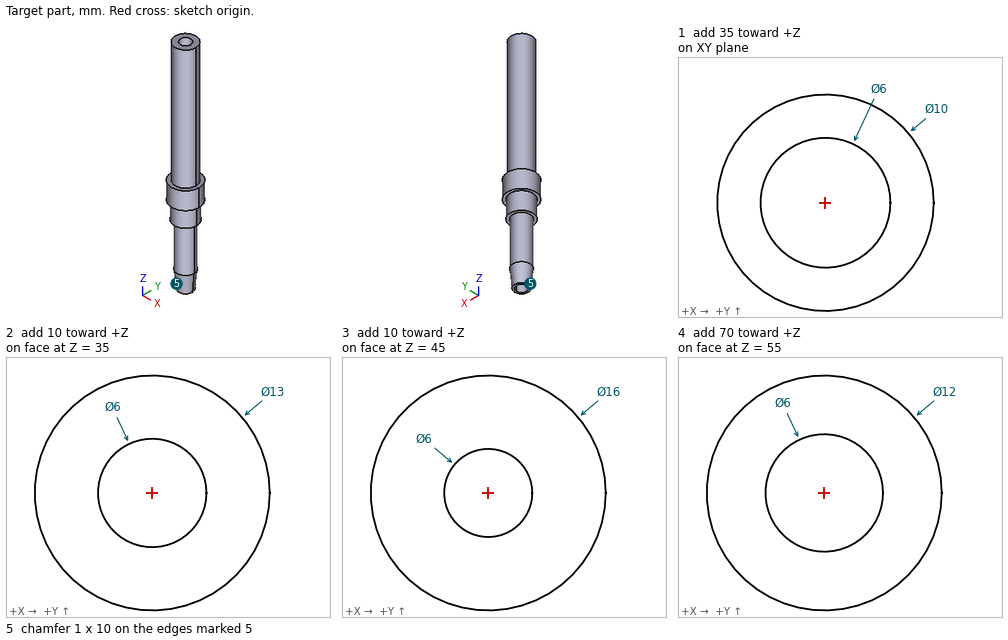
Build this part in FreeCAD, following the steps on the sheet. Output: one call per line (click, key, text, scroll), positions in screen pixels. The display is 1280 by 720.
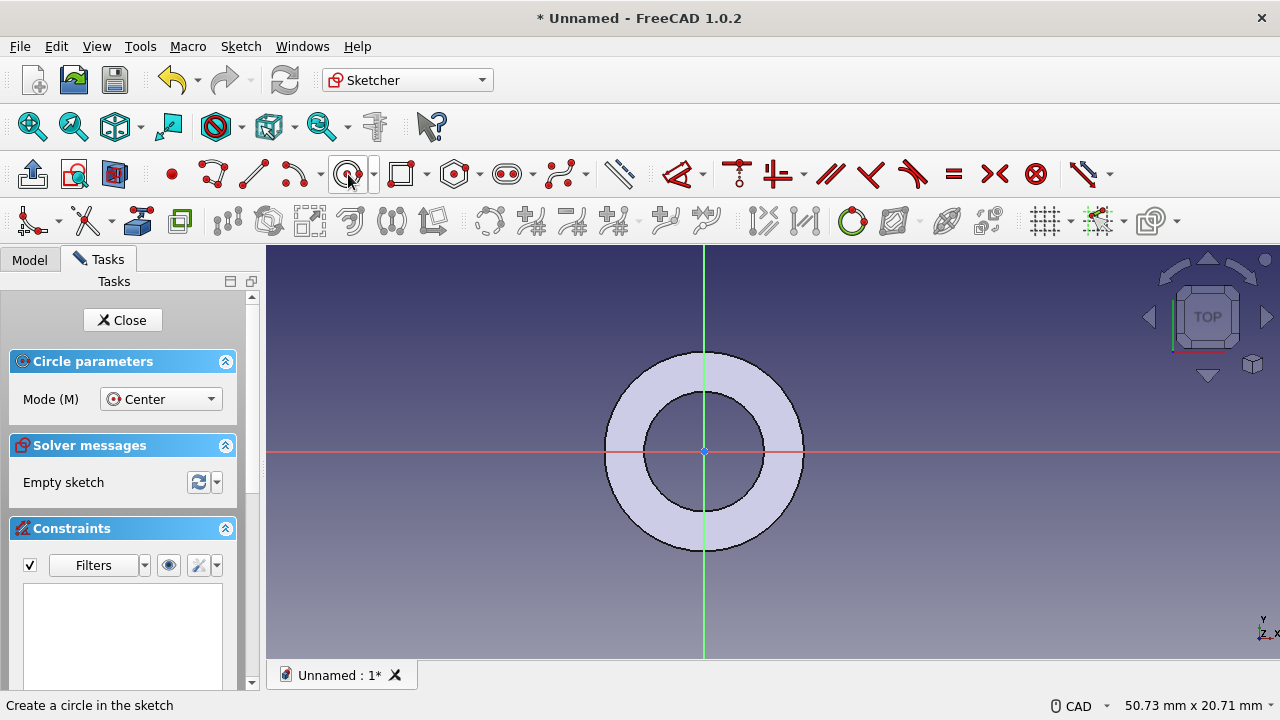
click(704, 452)
click(796, 360)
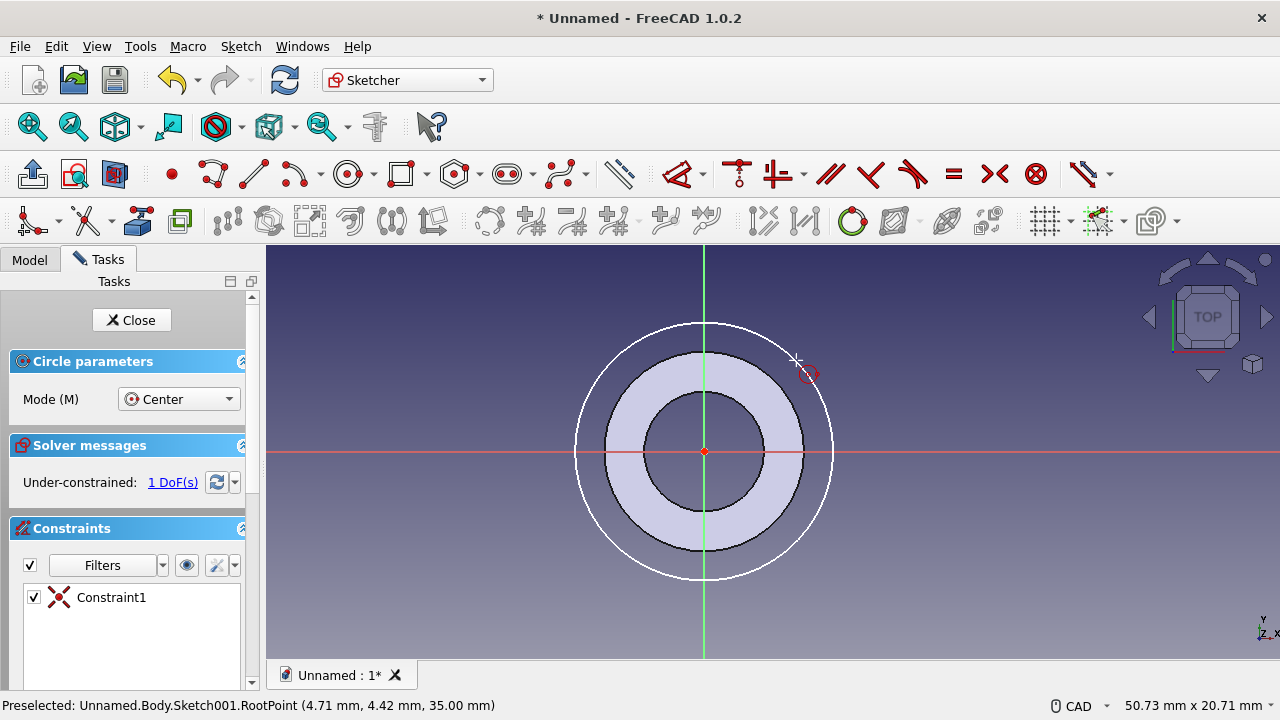
click(704, 452)
click(747, 409)
key(Escape)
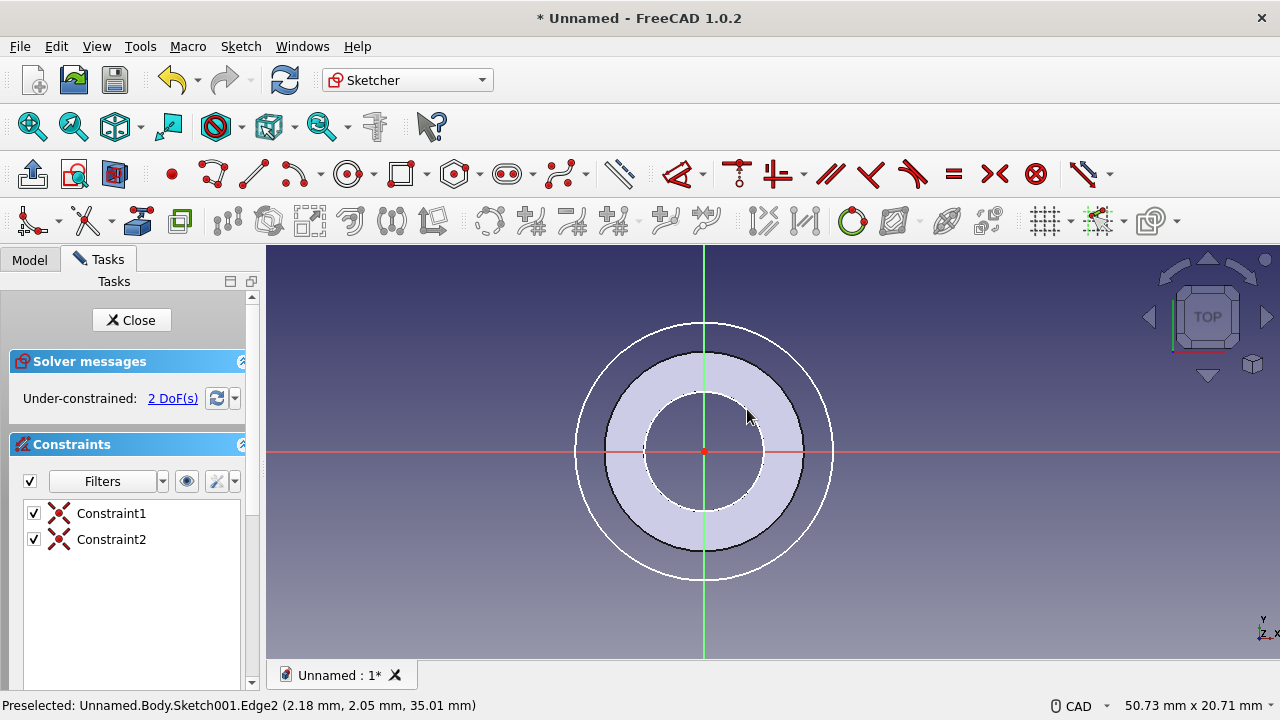
click(676, 174)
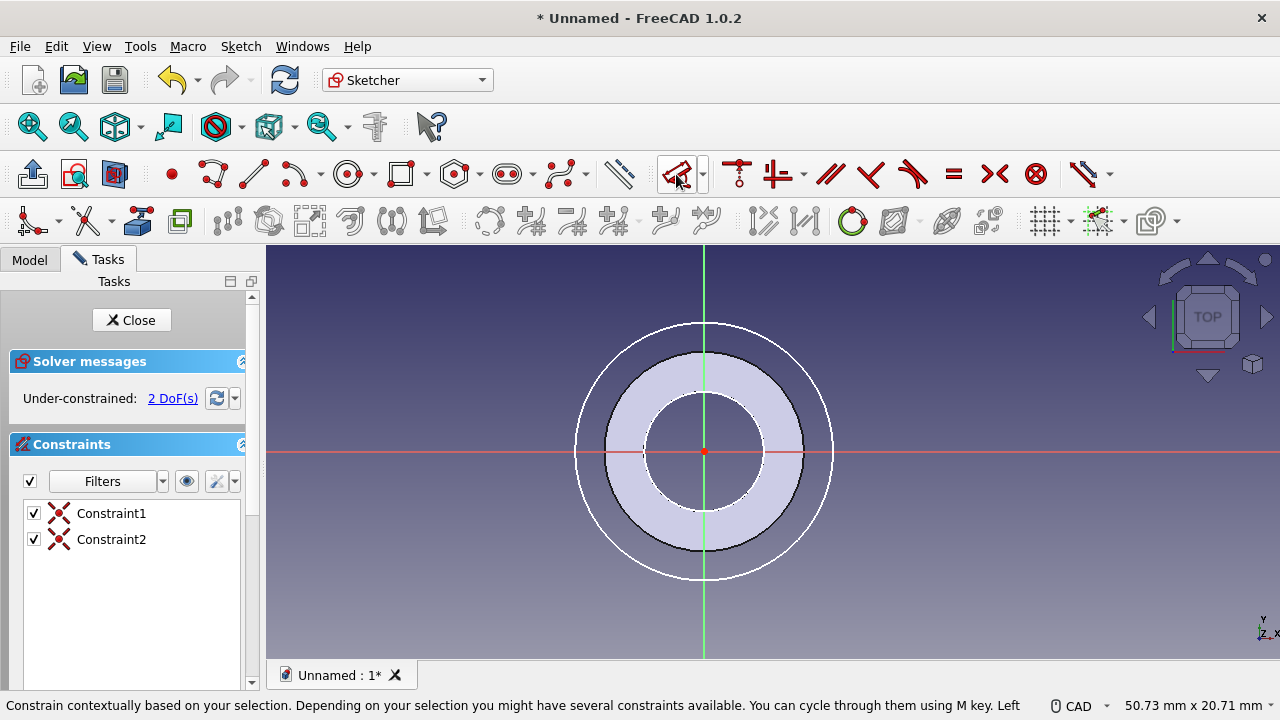
click(795, 360)
click(818, 337)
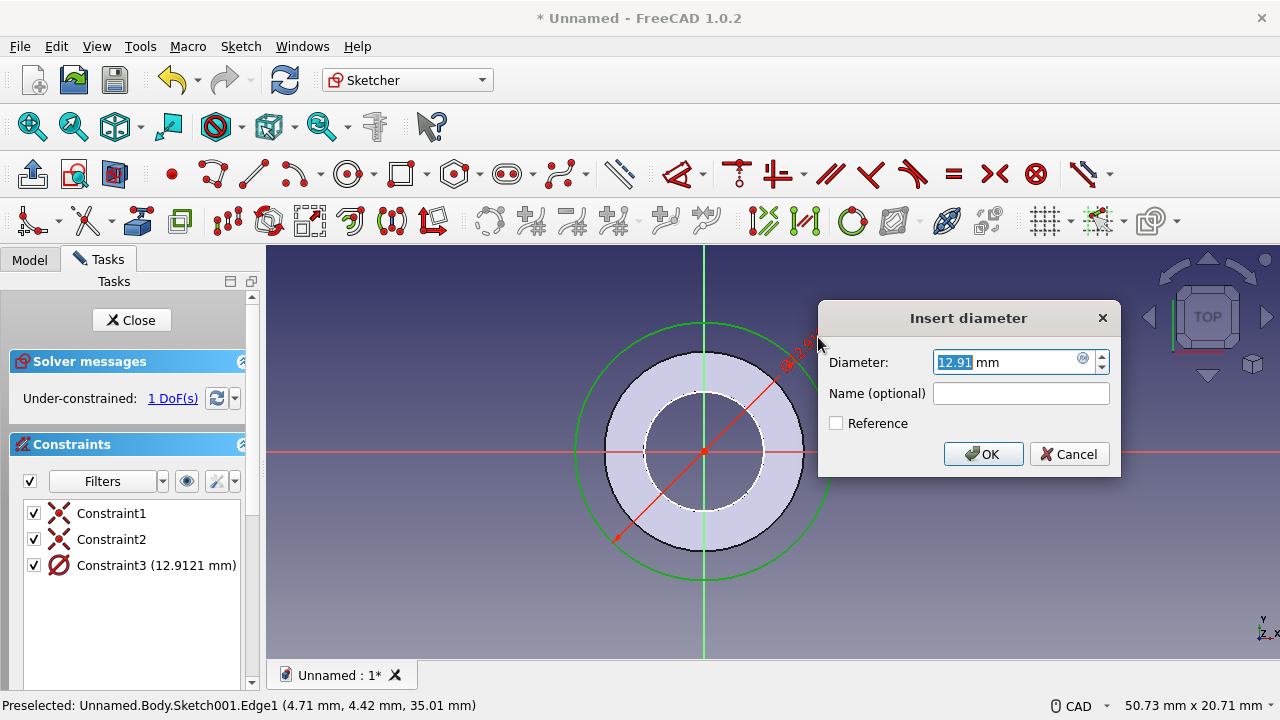
text(13)
key(Return)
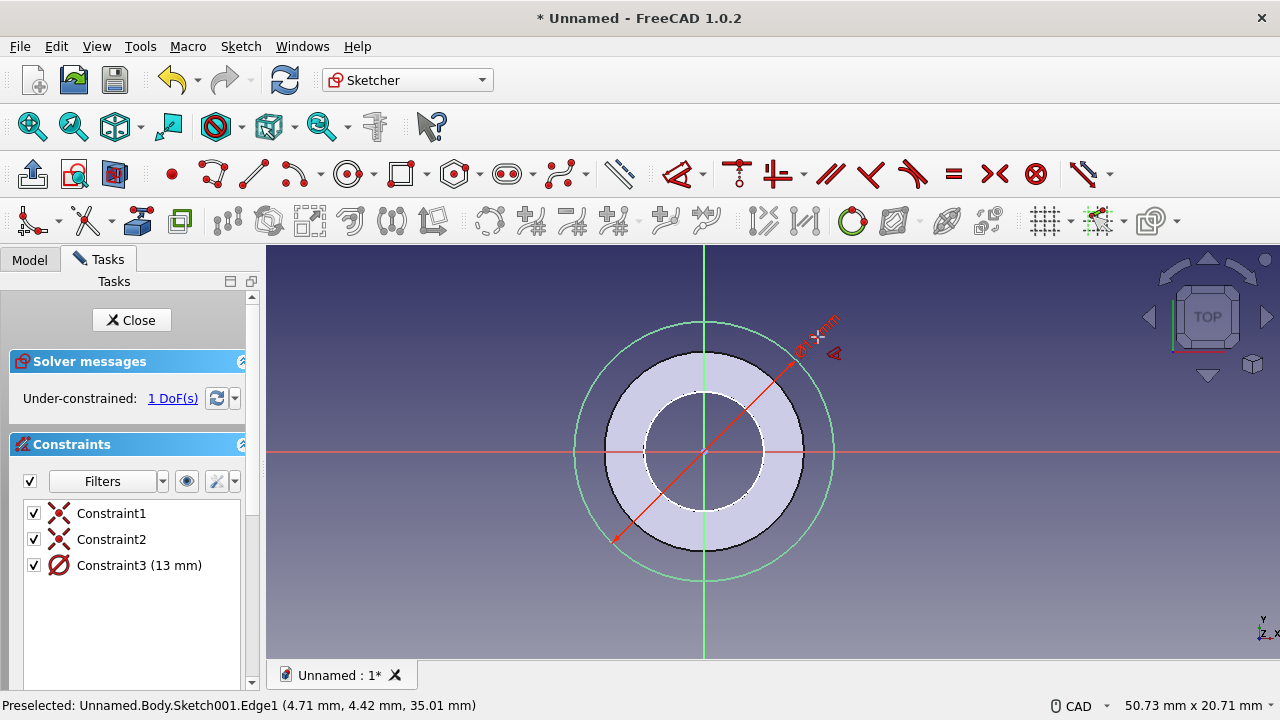
click(746, 409)
click(768, 386)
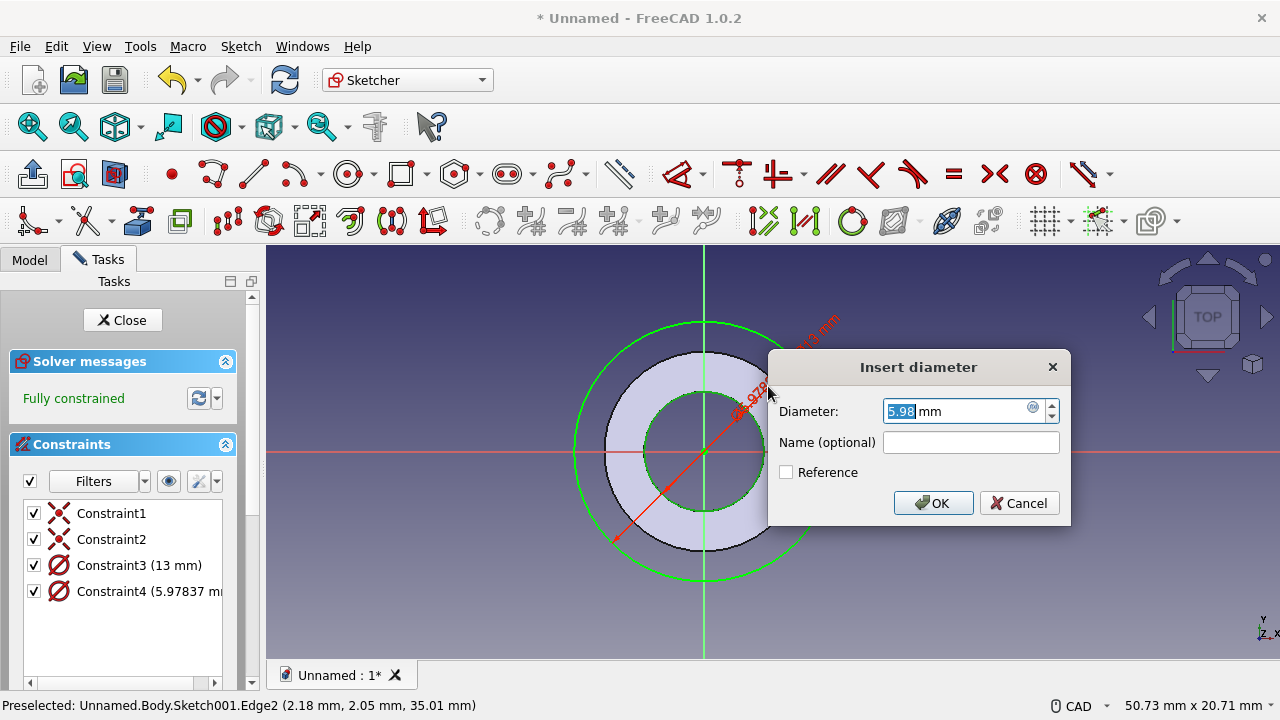
text(6)
key(Return)
key(Escape)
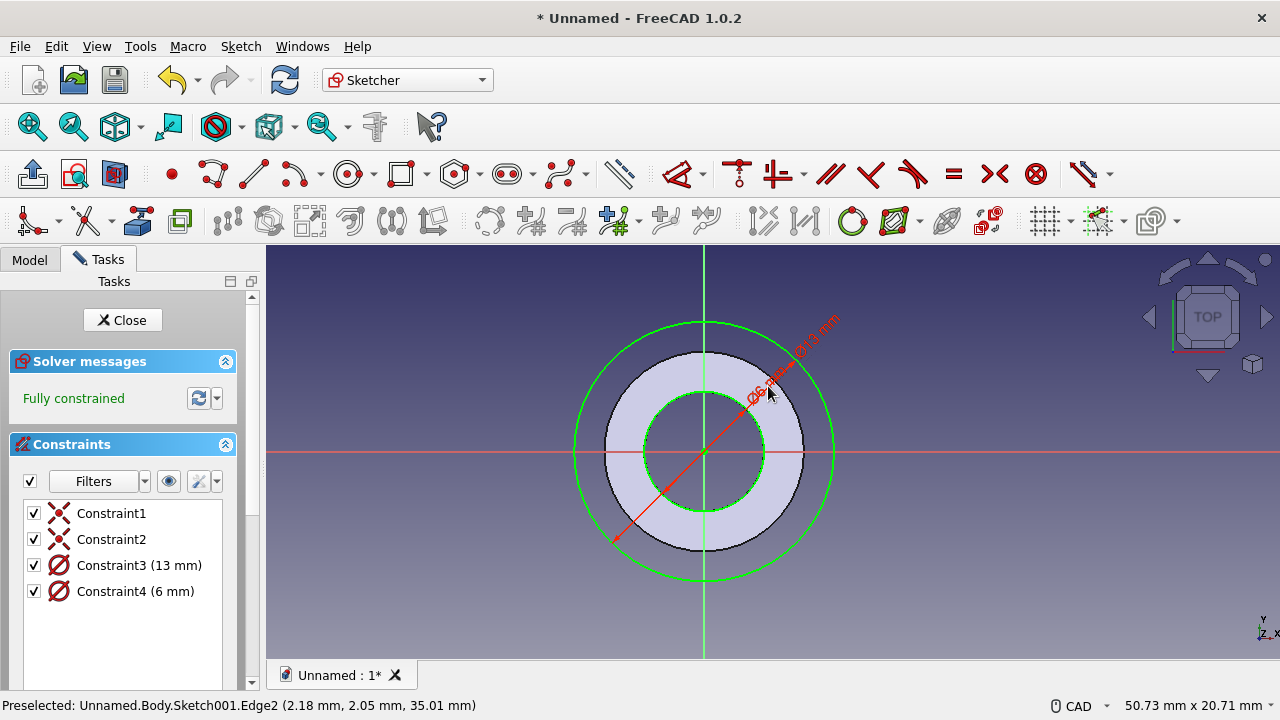
click(123, 320)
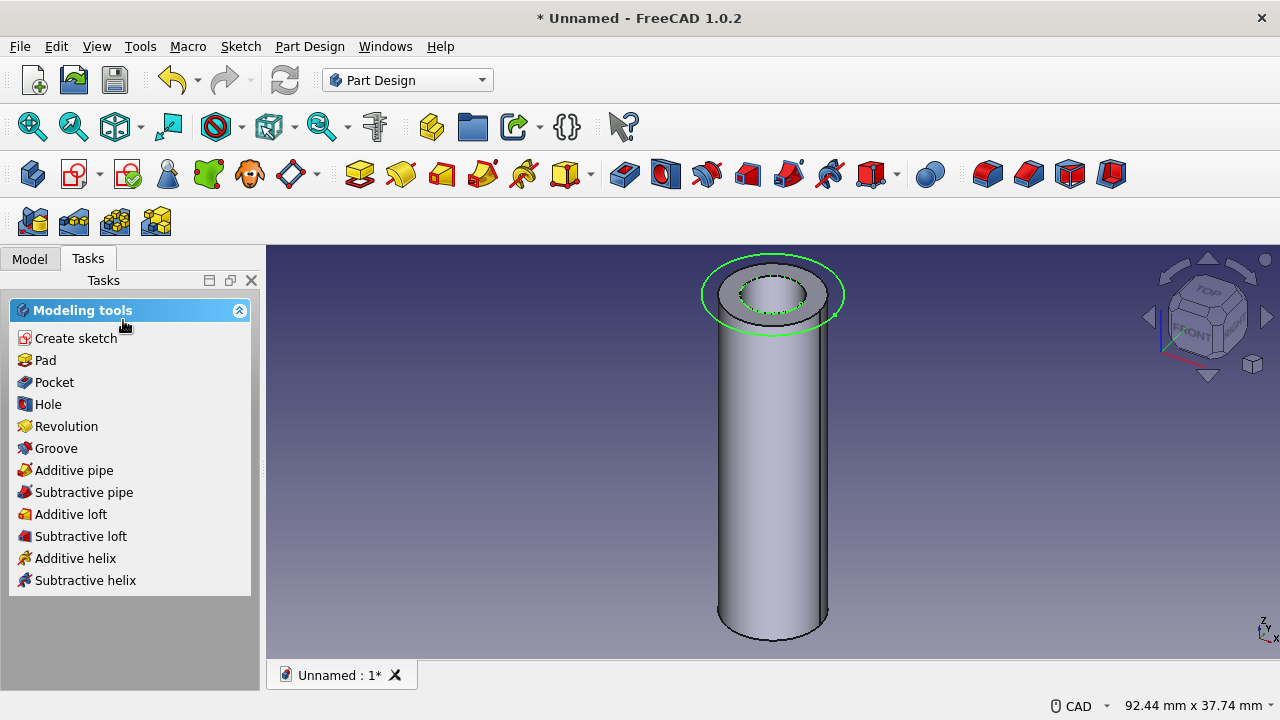
click(360, 174)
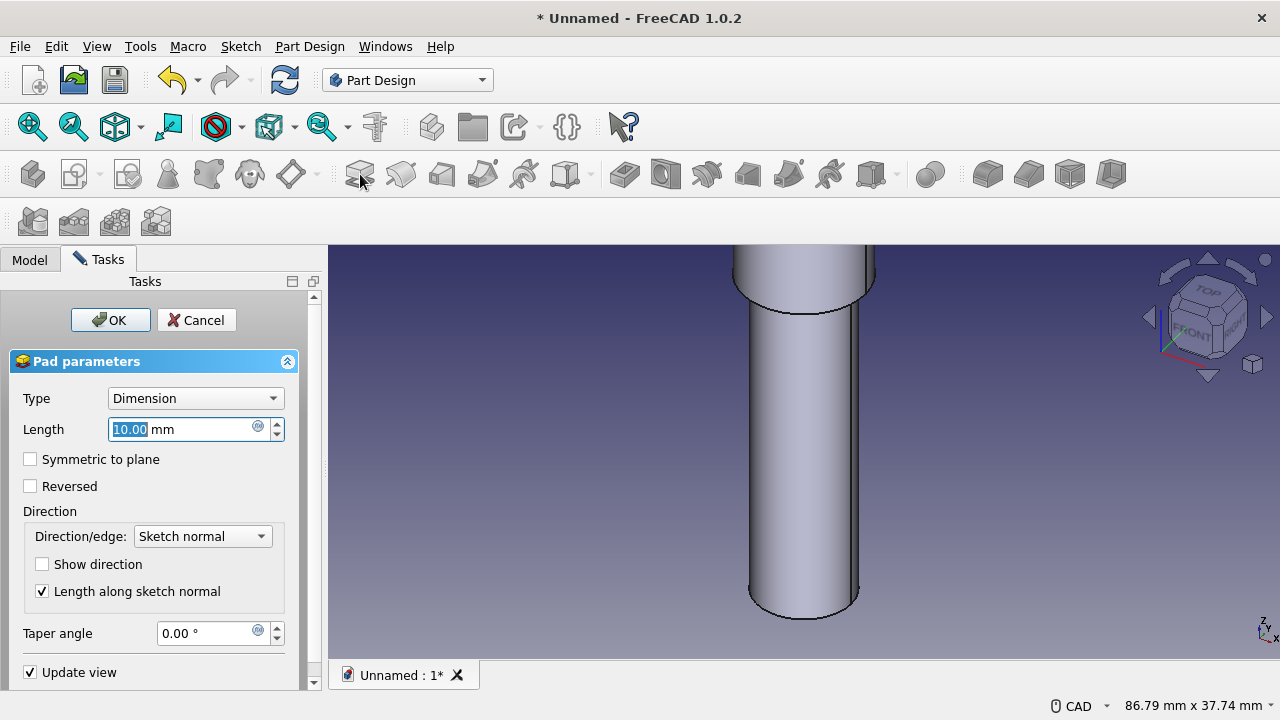
text(10)
key(Tab)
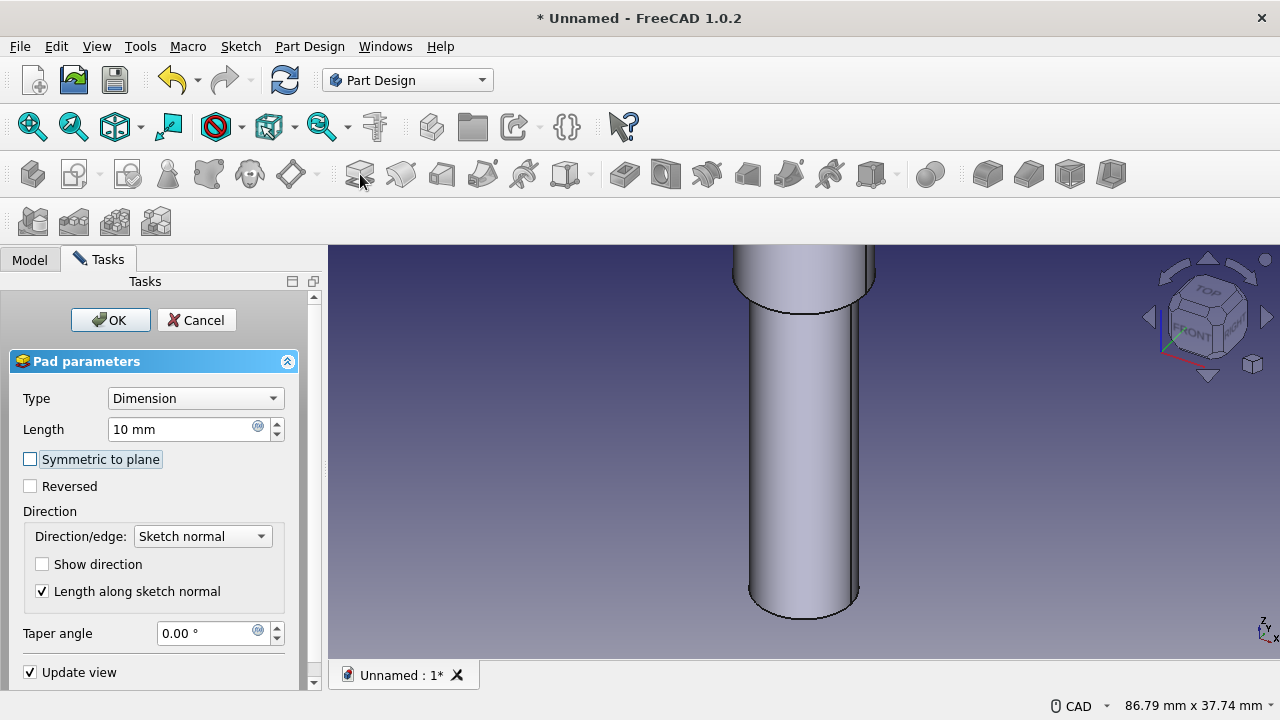
click(111, 320)